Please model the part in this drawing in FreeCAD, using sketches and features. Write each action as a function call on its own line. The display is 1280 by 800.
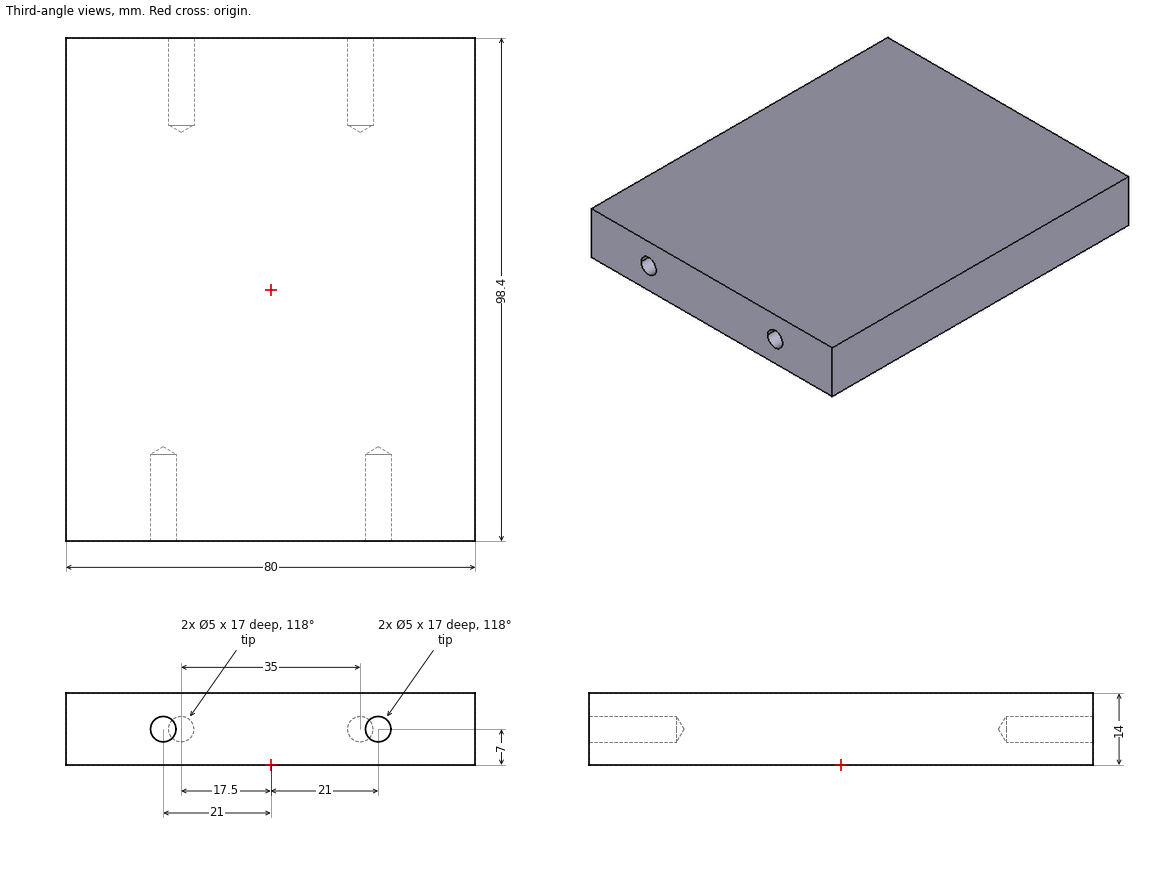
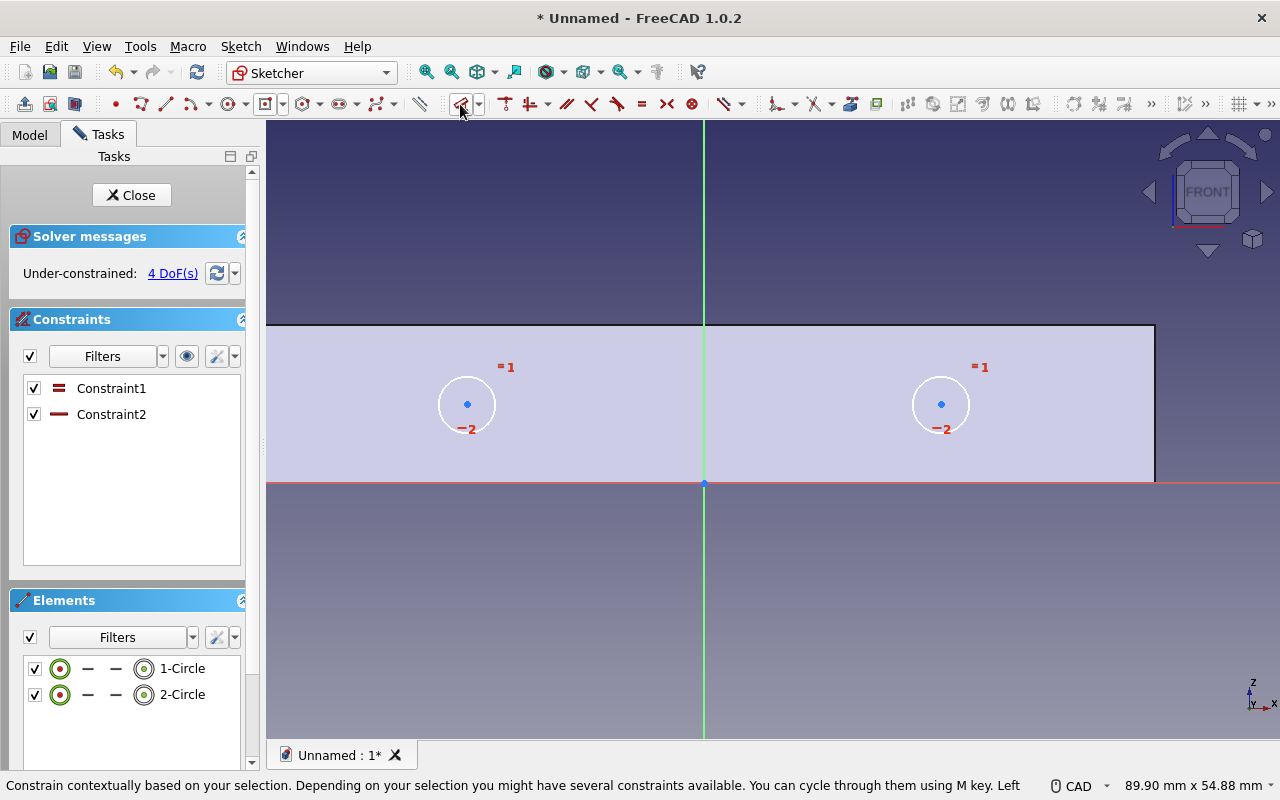
click(961, 385)
click(984, 362)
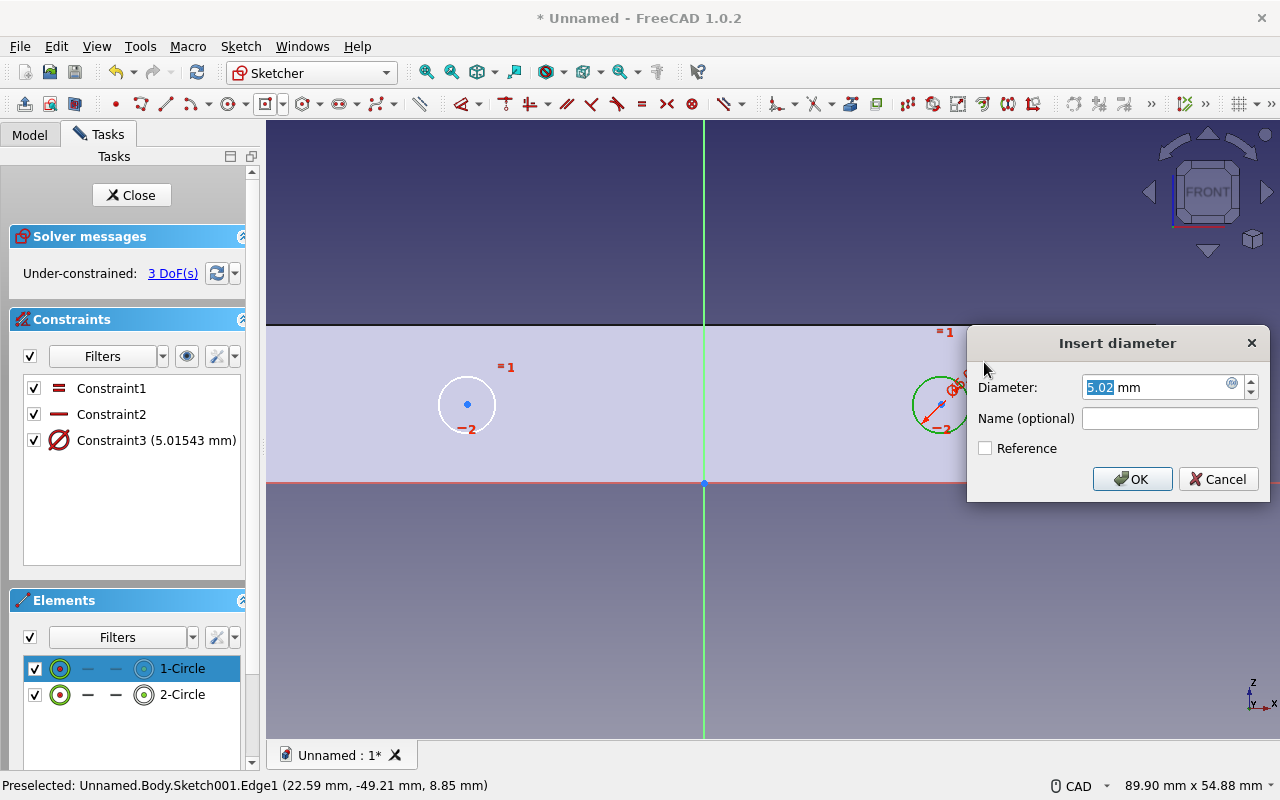
text(5)
key(Return)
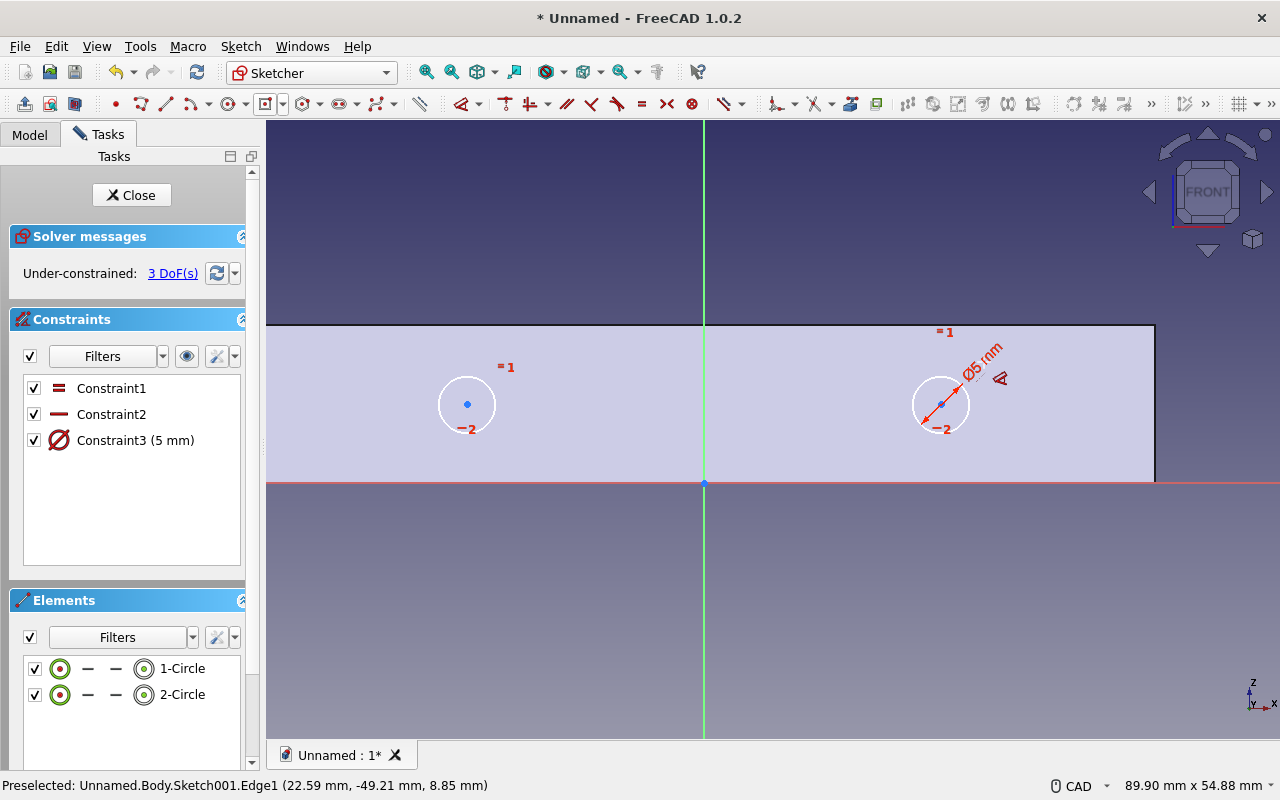
click(941, 405)
click(975, 444)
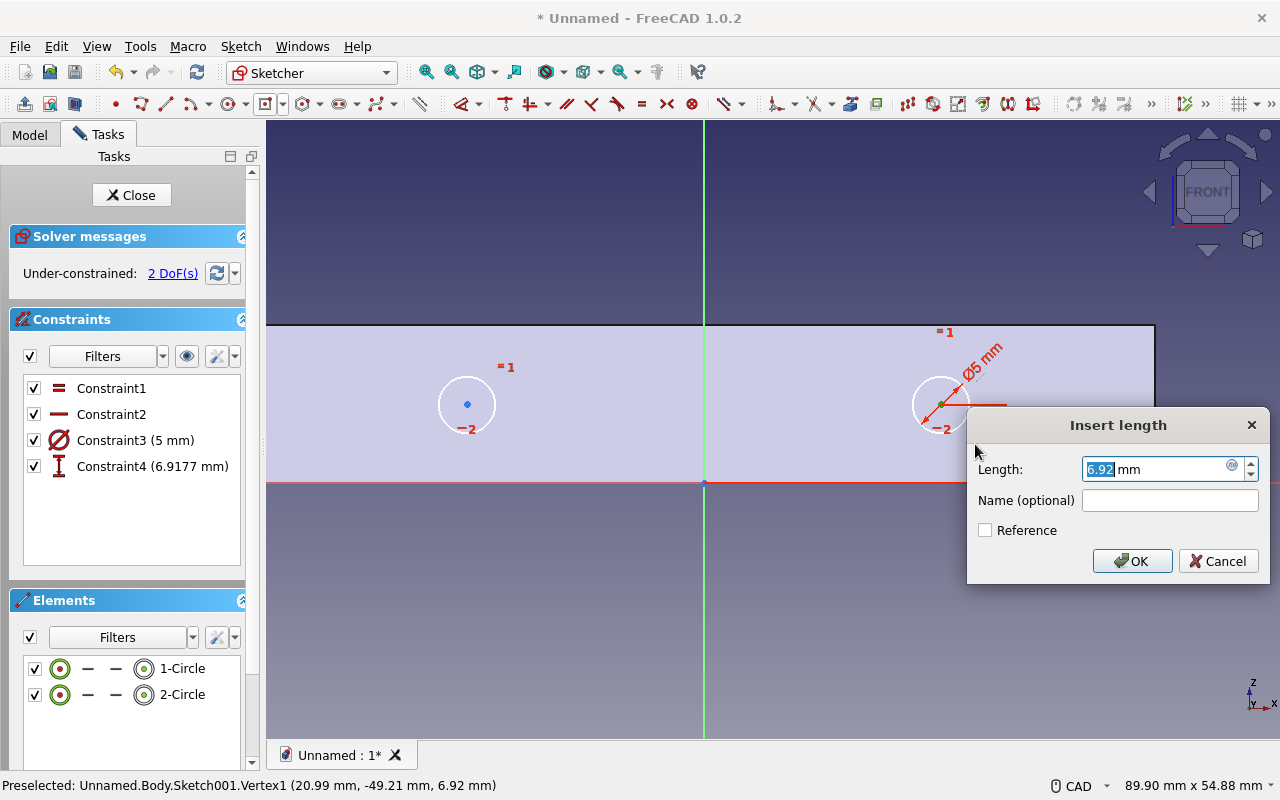
text(7)
key(Return)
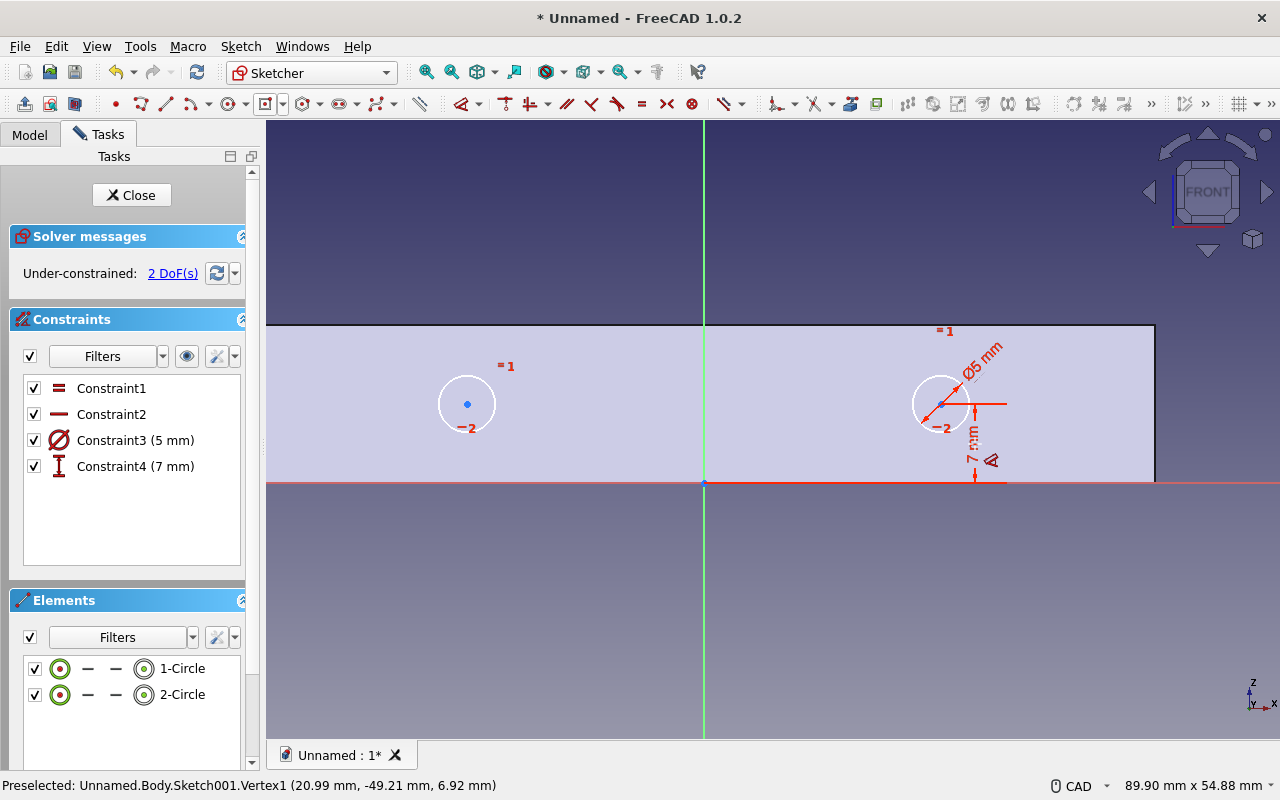
click(941, 404)
click(823, 517)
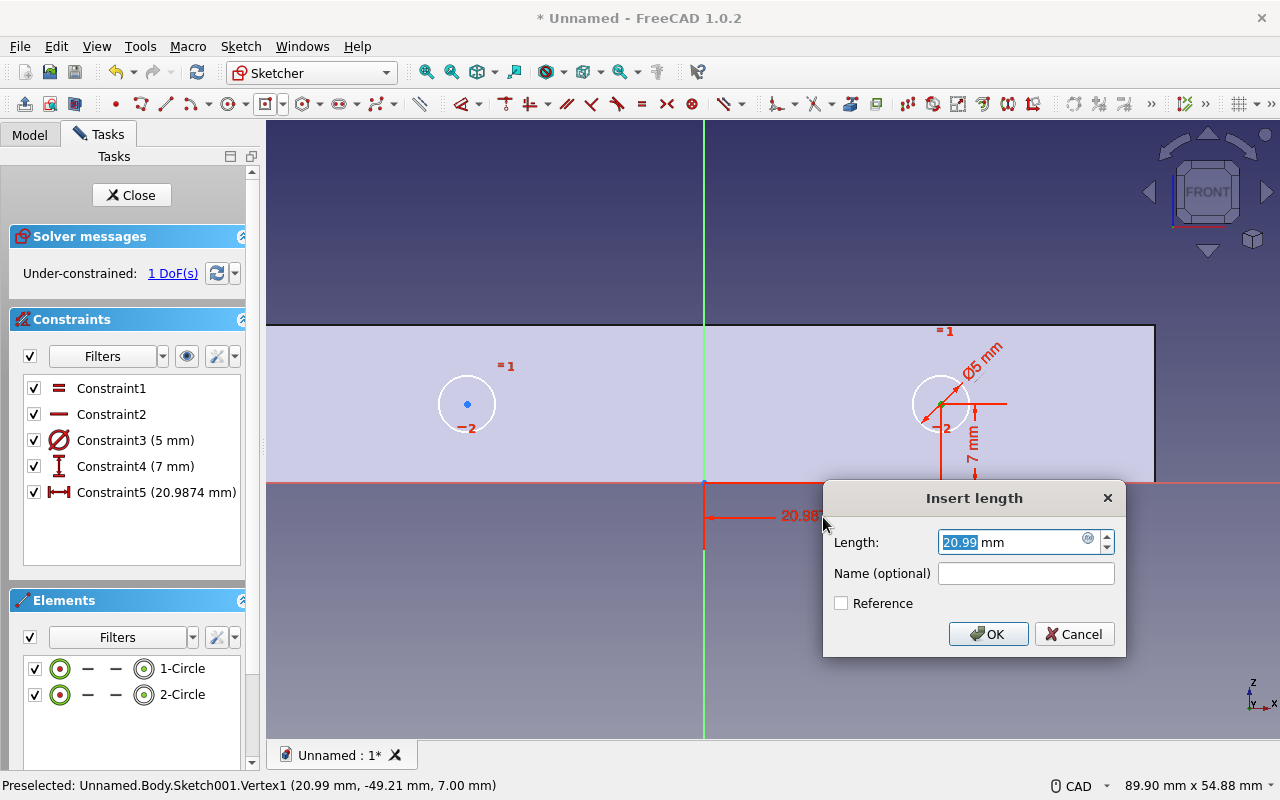
text(21)
key(Return)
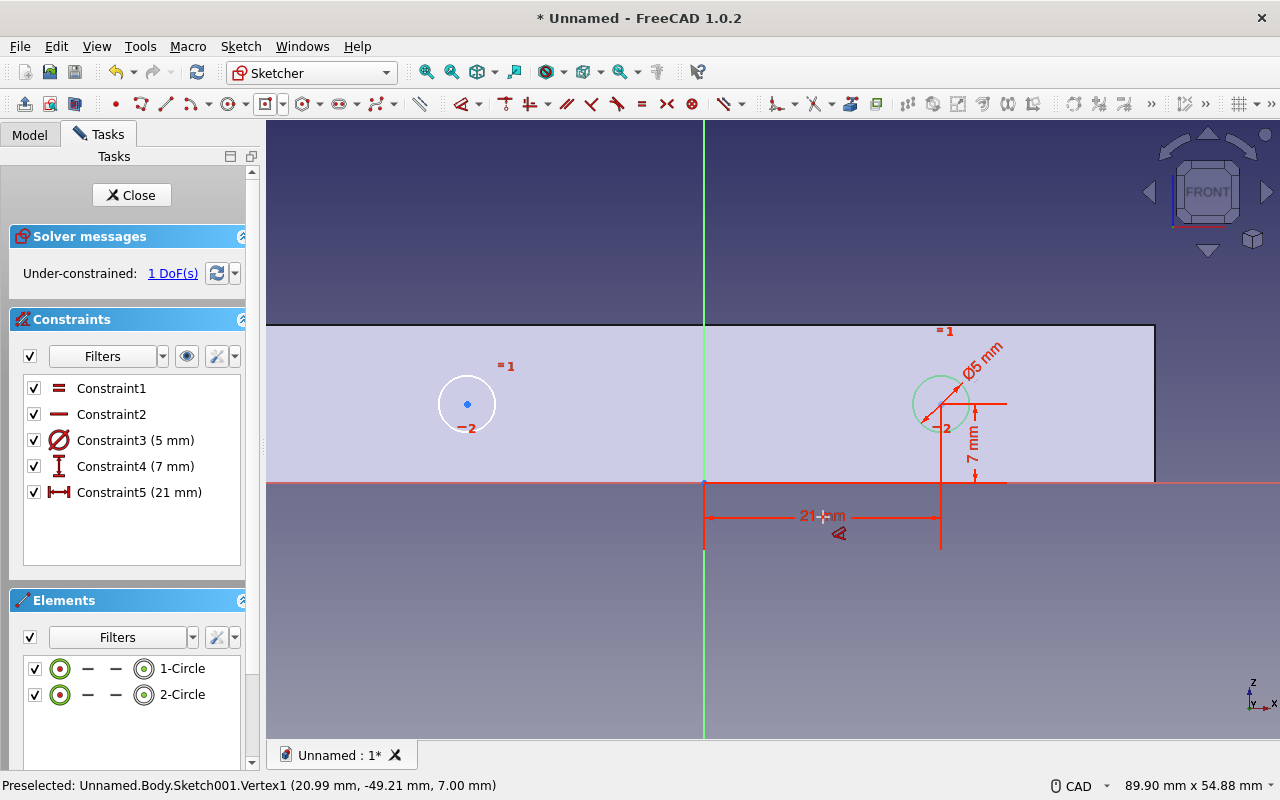
click(467, 404)
click(586, 517)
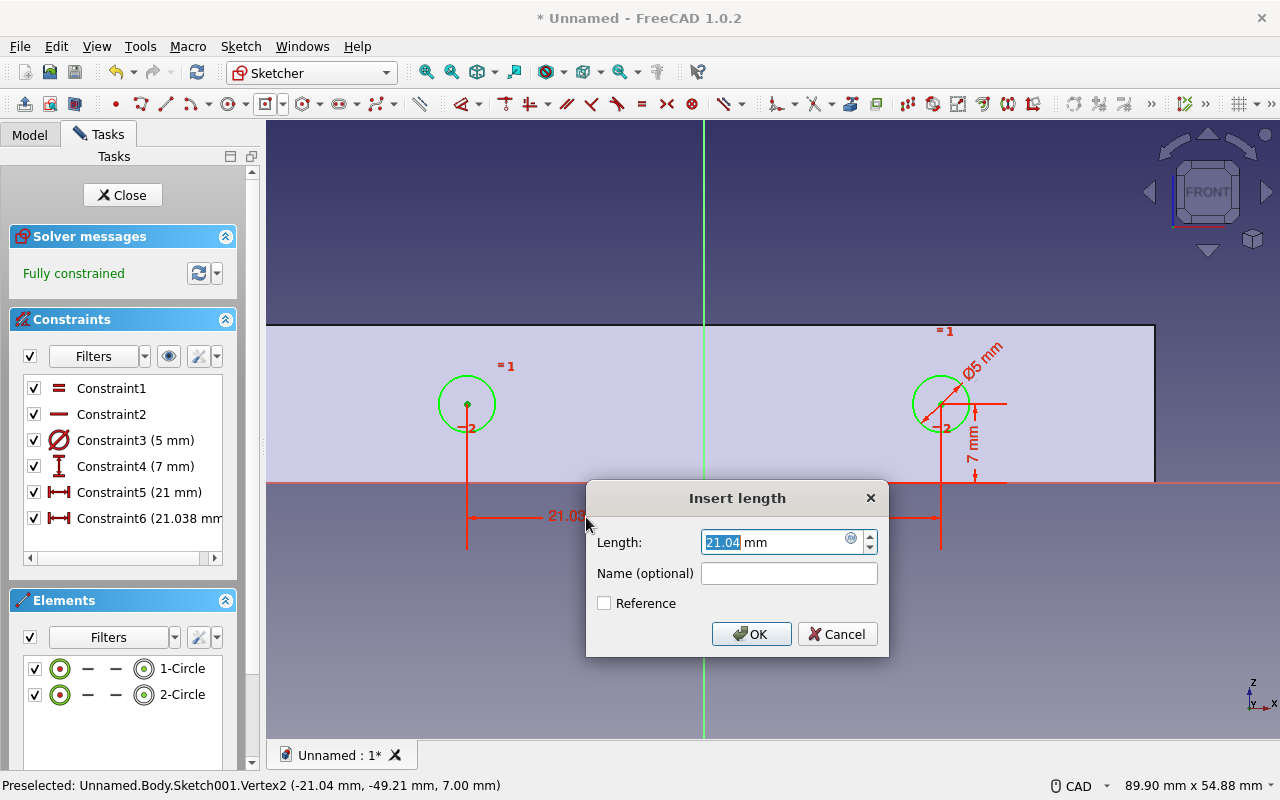
text(21)
key(Return)
key(Escape)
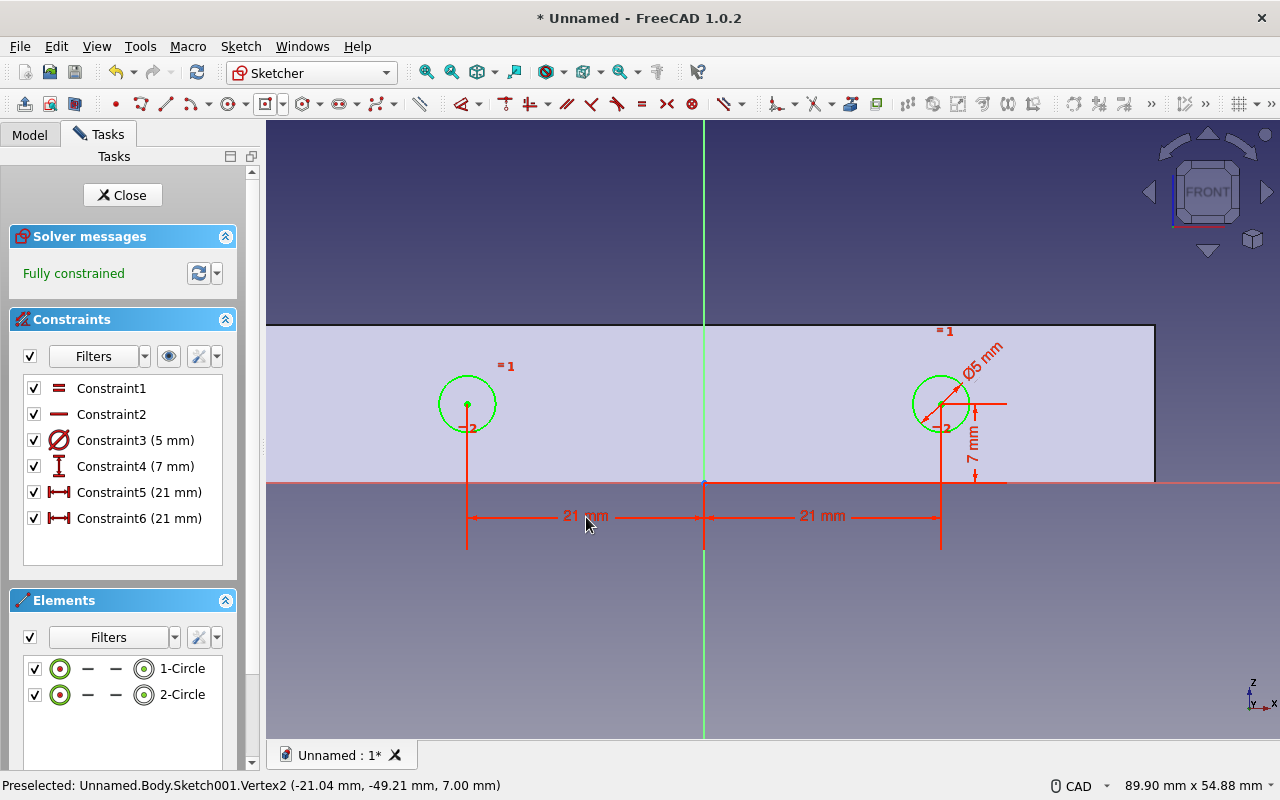
click(123, 195)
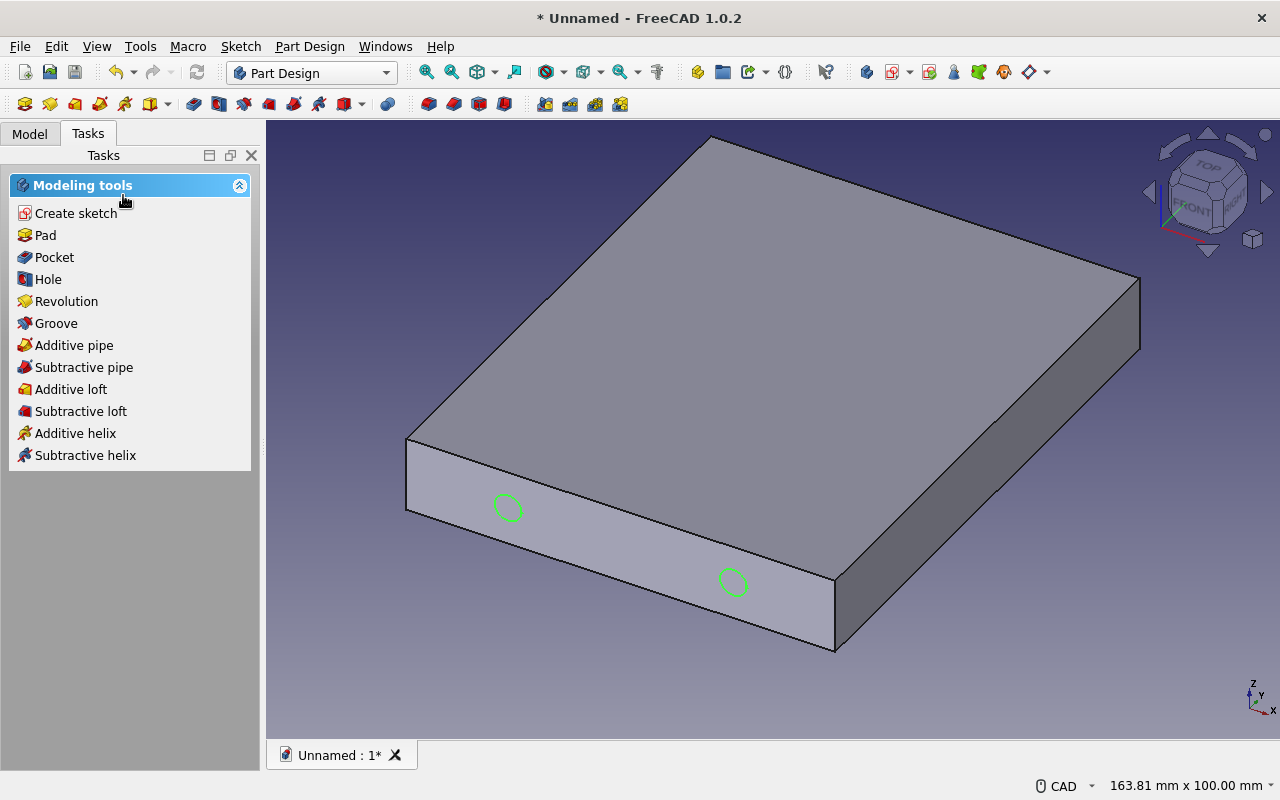
click(219, 104)